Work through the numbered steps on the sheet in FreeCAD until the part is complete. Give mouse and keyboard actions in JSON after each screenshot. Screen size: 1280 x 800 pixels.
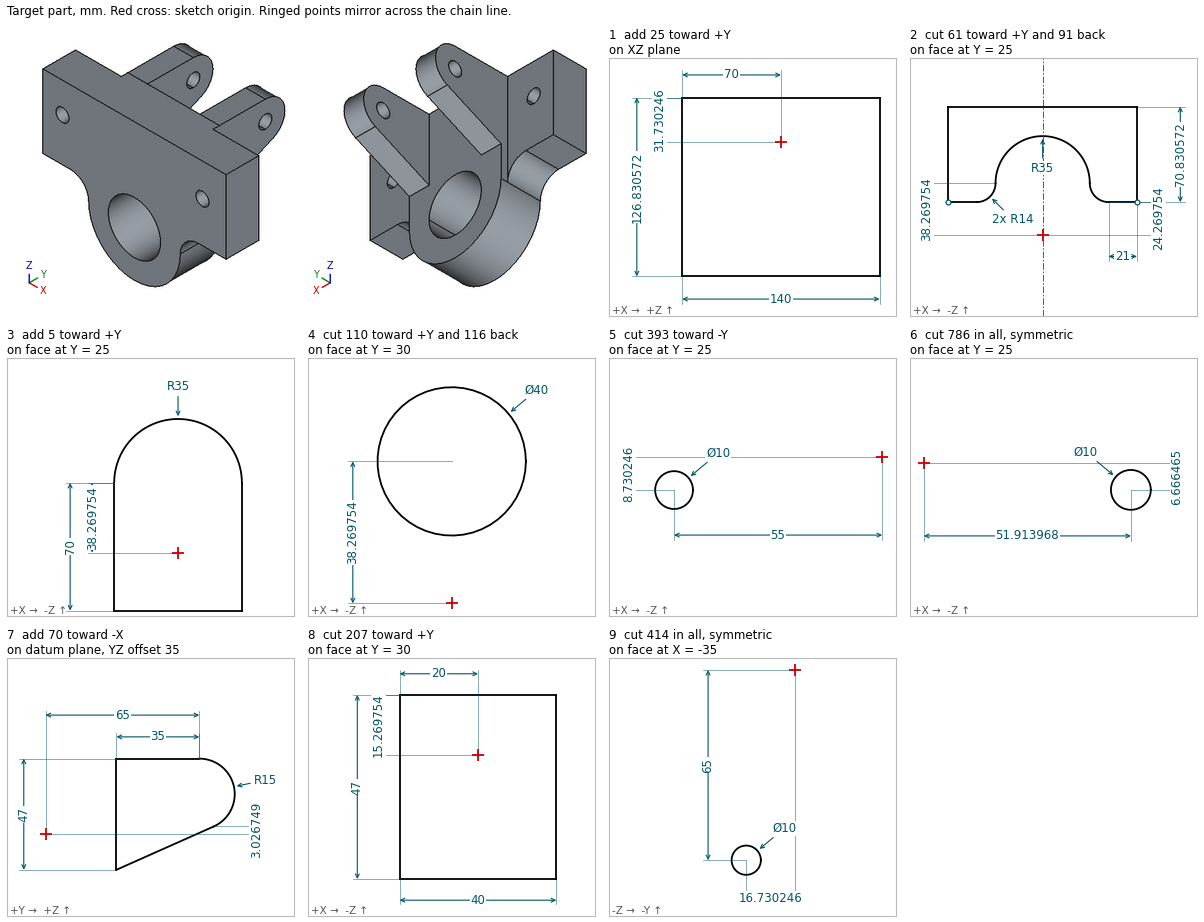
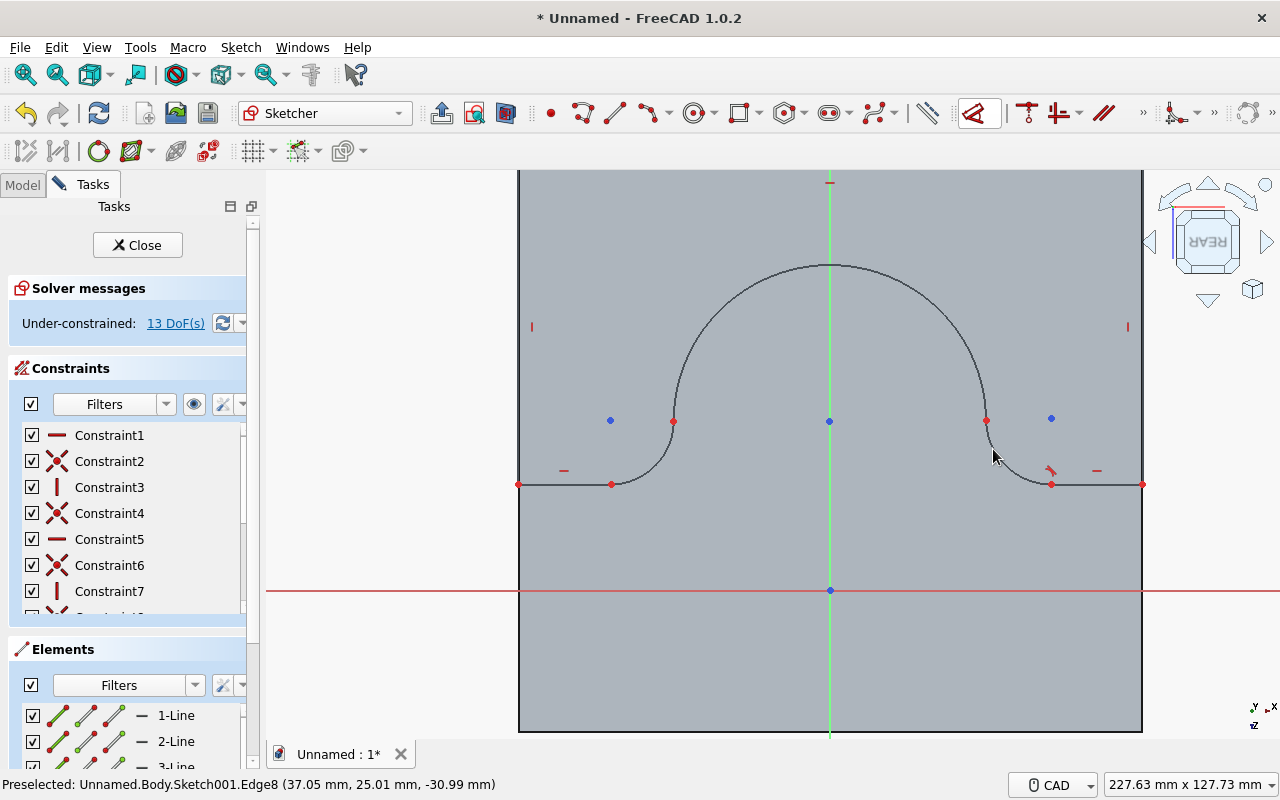
{"action": "left_click", "coordinate": [546, 485]}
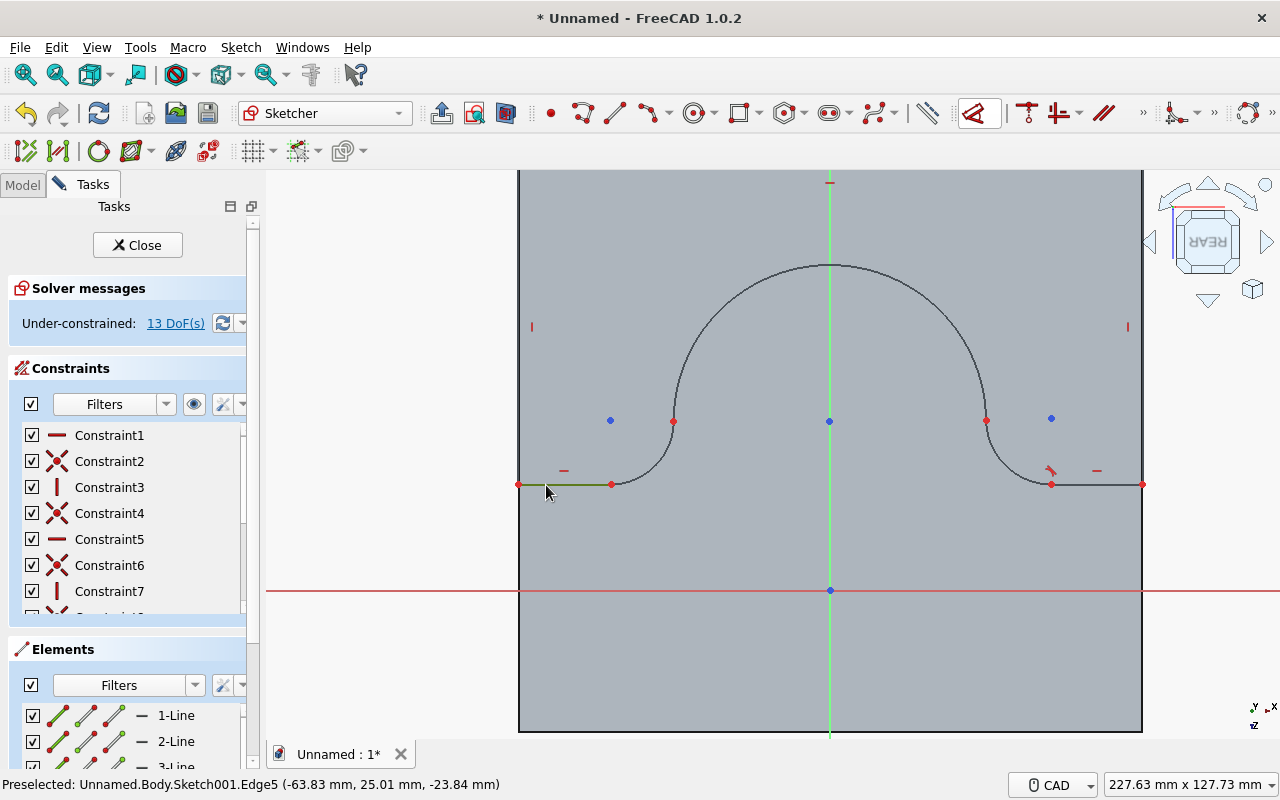
{"action": "left_click", "coordinate": [640, 477]}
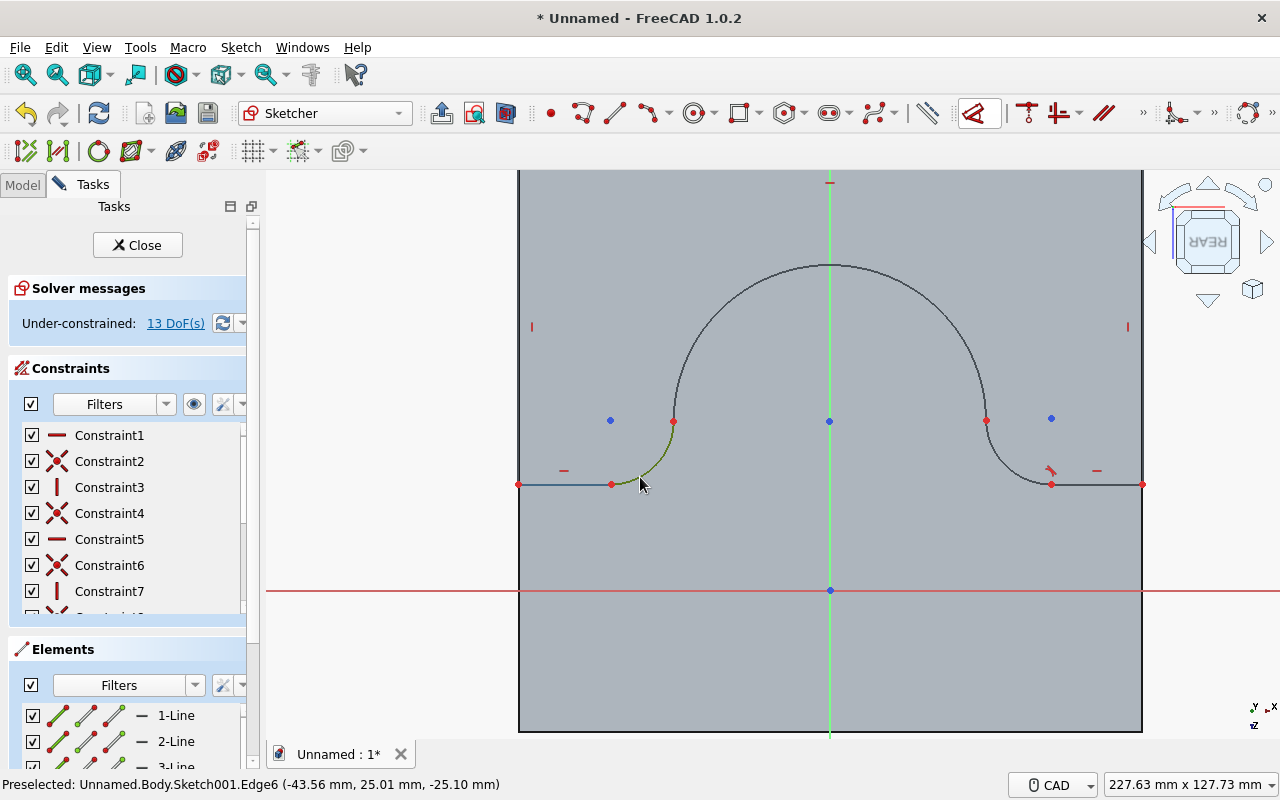
{"action": "key", "text": "t"}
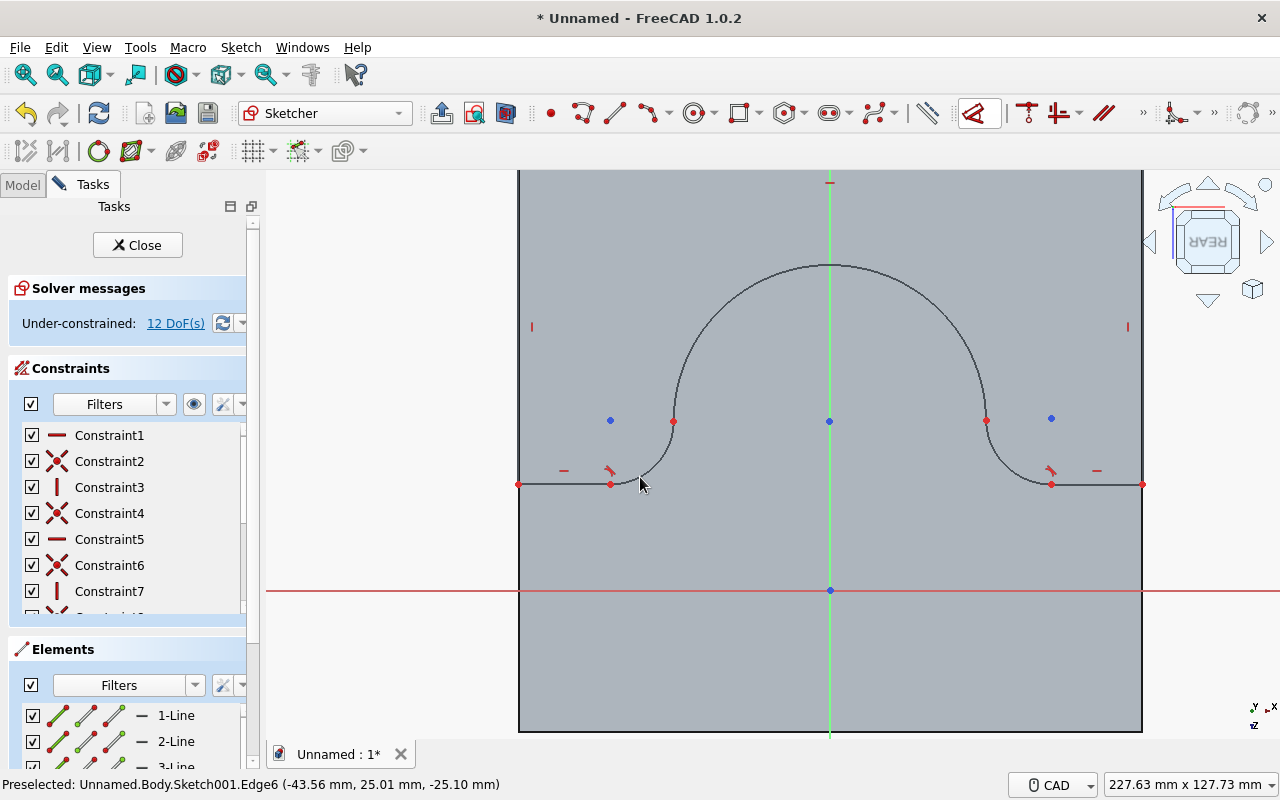
{"action": "left_click", "coordinate": [639, 478]}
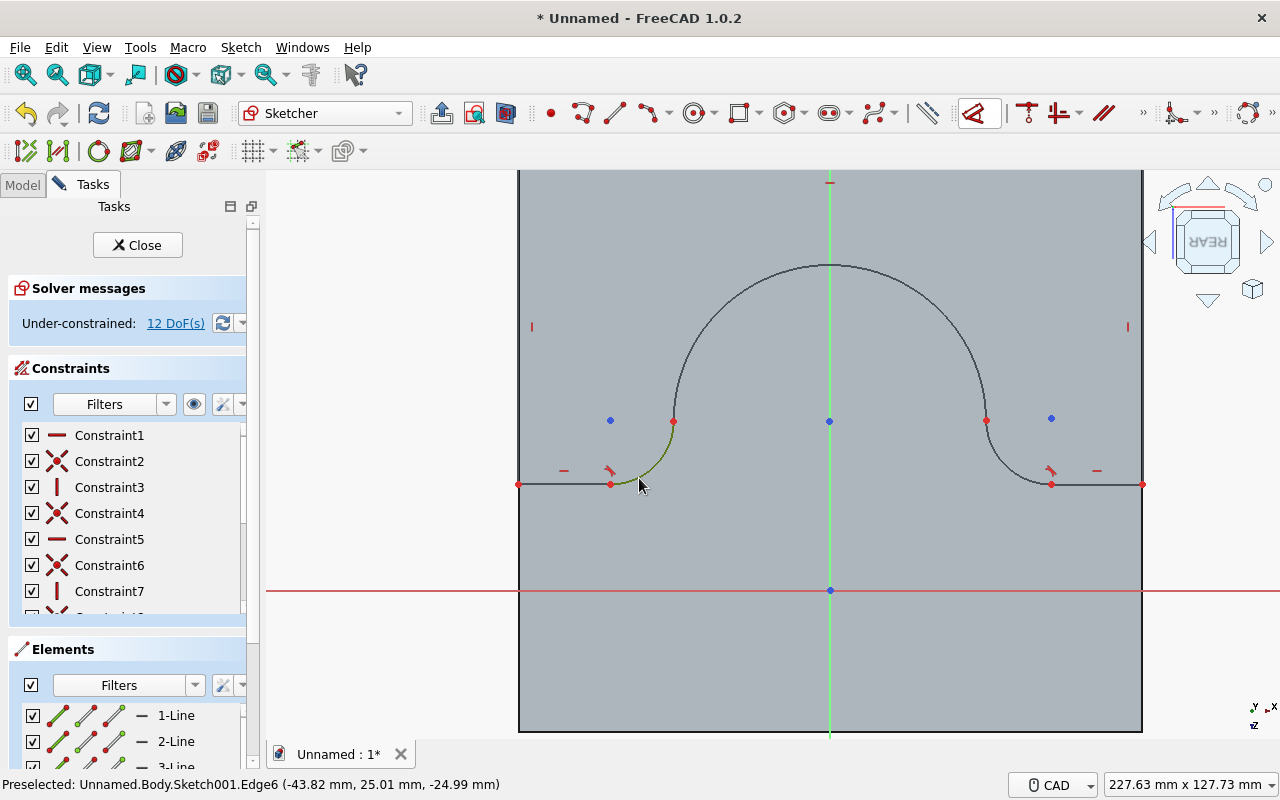
{"action": "left_click", "coordinate": [921, 295]}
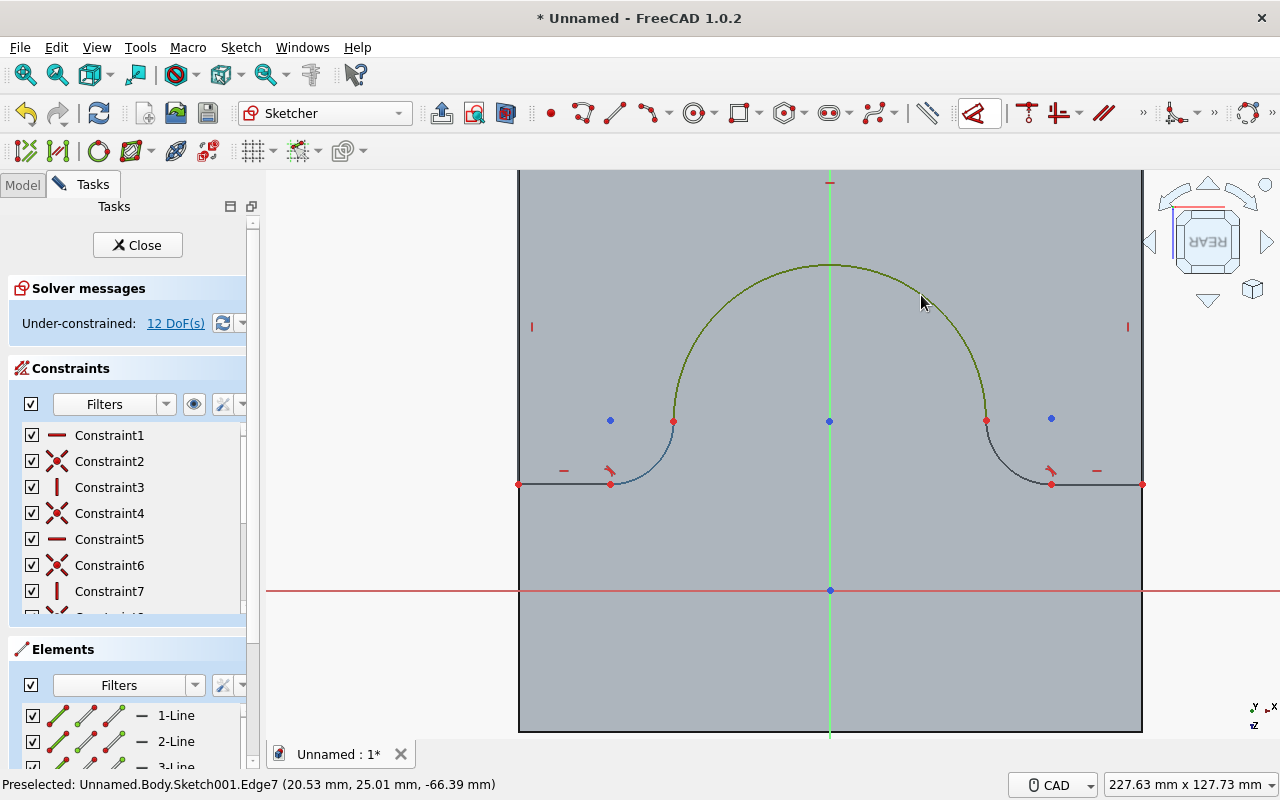
{"action": "key", "text": "t"}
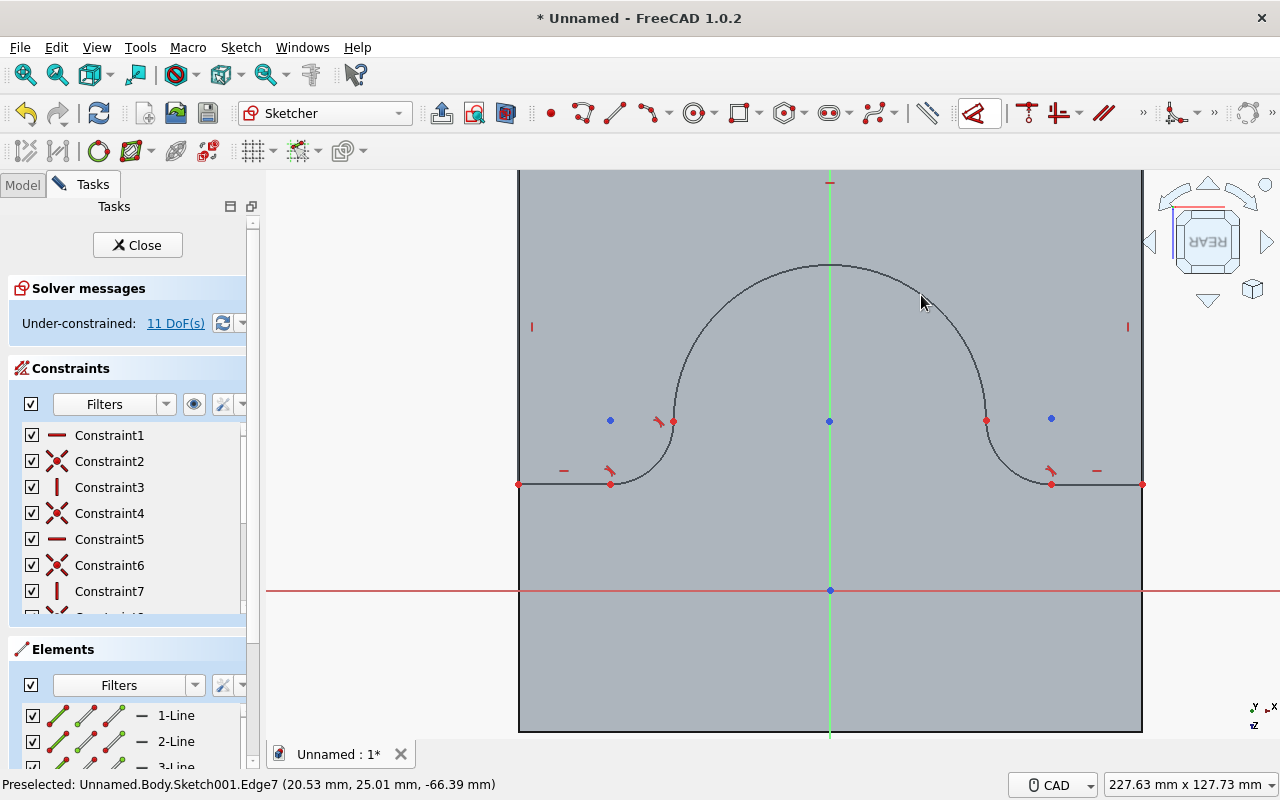
{"action": "left_click", "coordinate": [922, 295]}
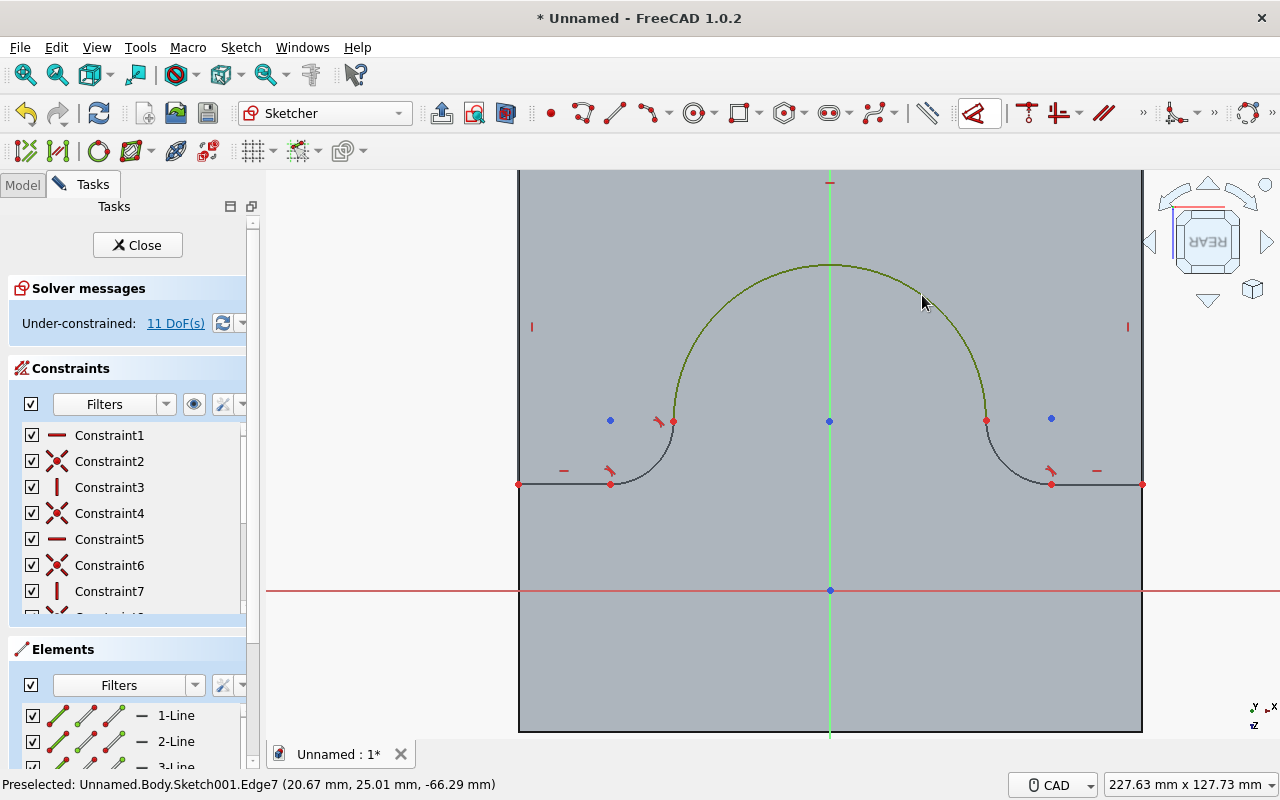
{"action": "left_click", "coordinate": [994, 450]}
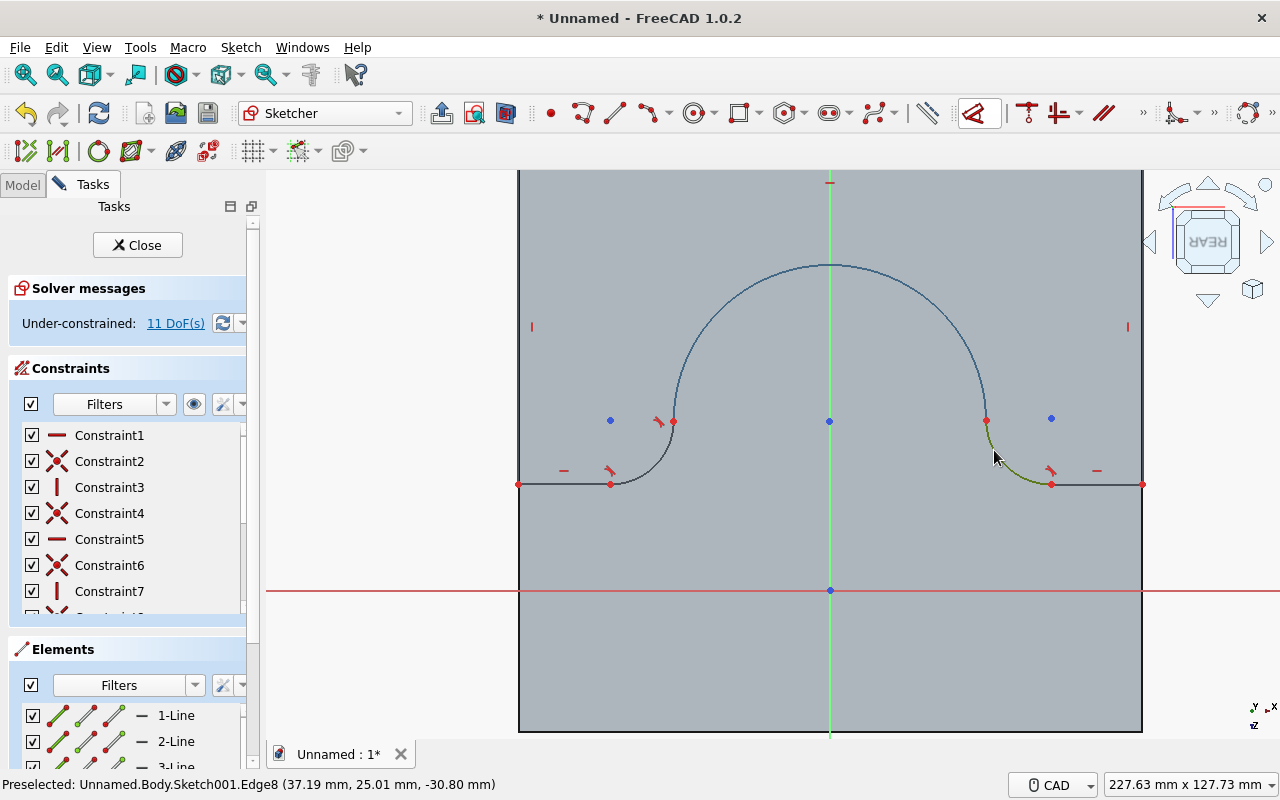
{"action": "key", "text": "t"}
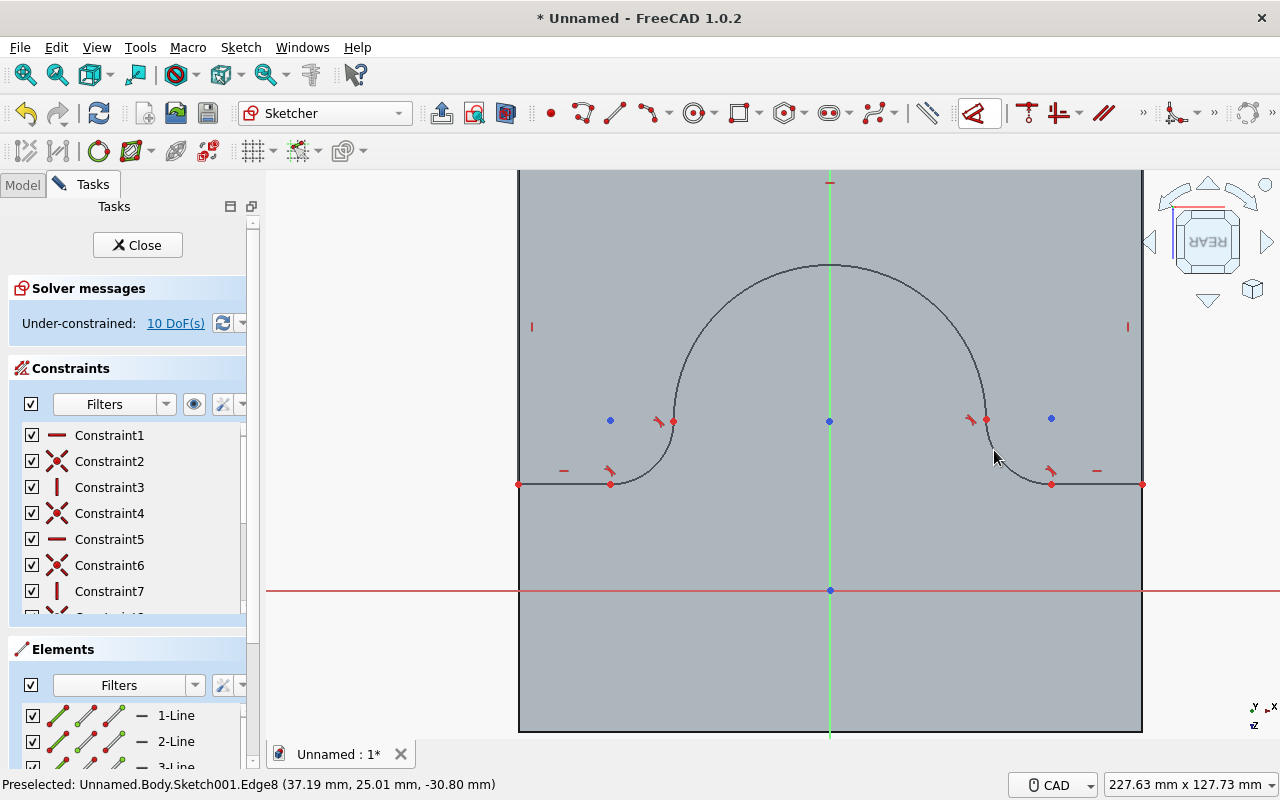
{"action": "left_click", "coordinate": [639, 478]}